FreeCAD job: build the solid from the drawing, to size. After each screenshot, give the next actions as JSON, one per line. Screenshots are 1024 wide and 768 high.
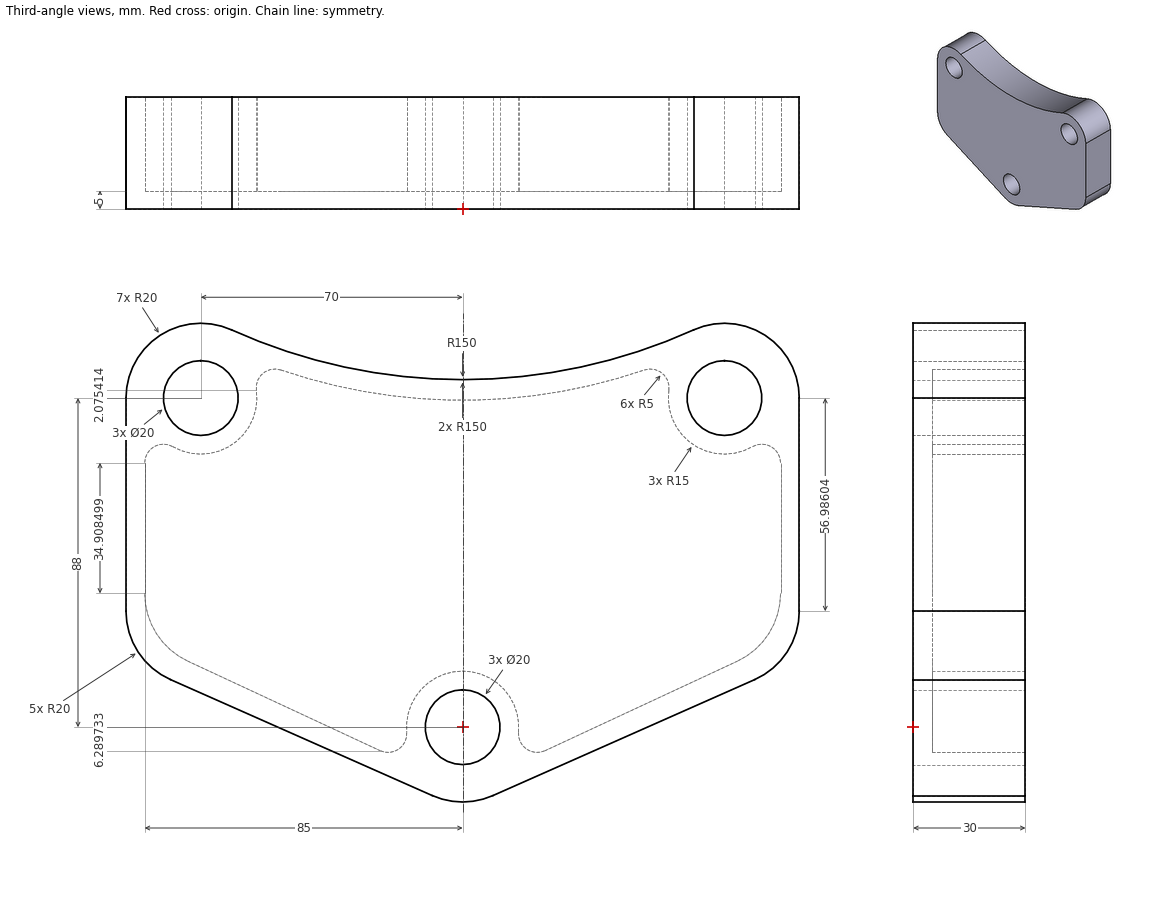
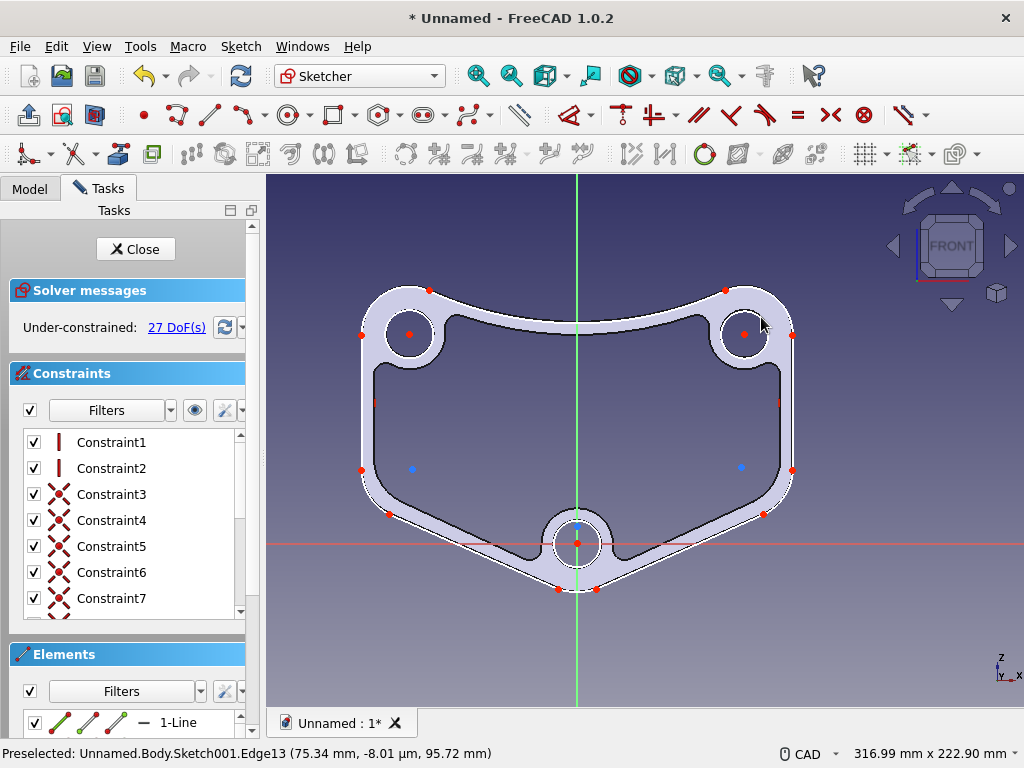
{"action": "left_click", "coordinate": [362, 376]}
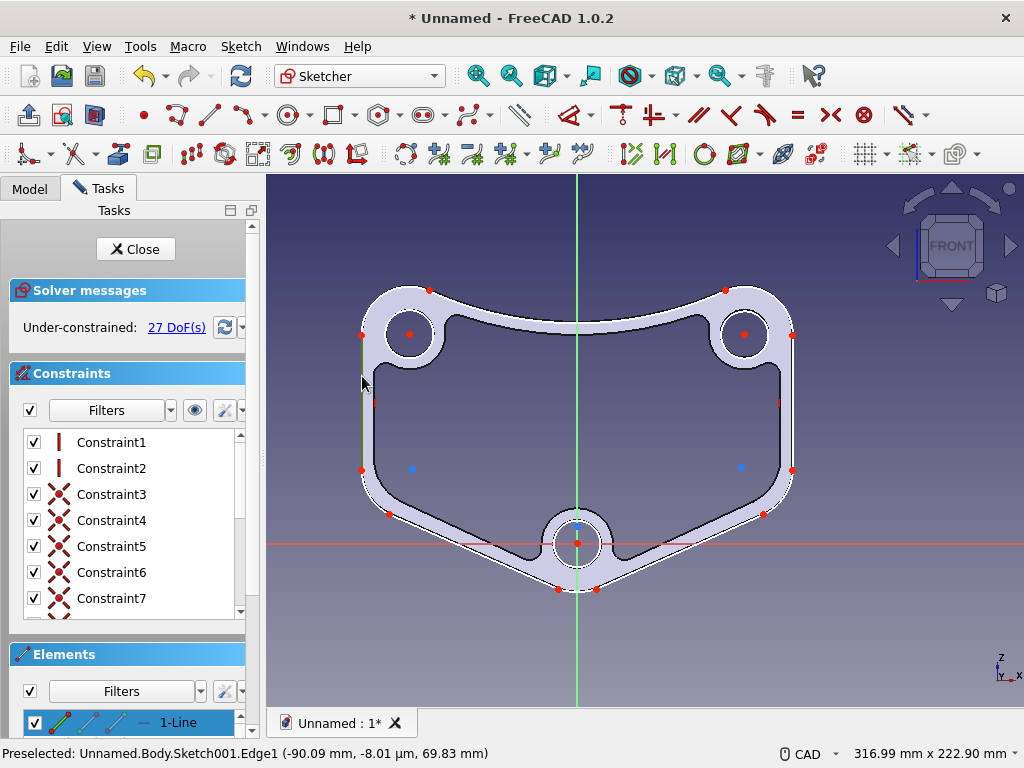
{"action": "left_click", "coordinate": [365, 487]}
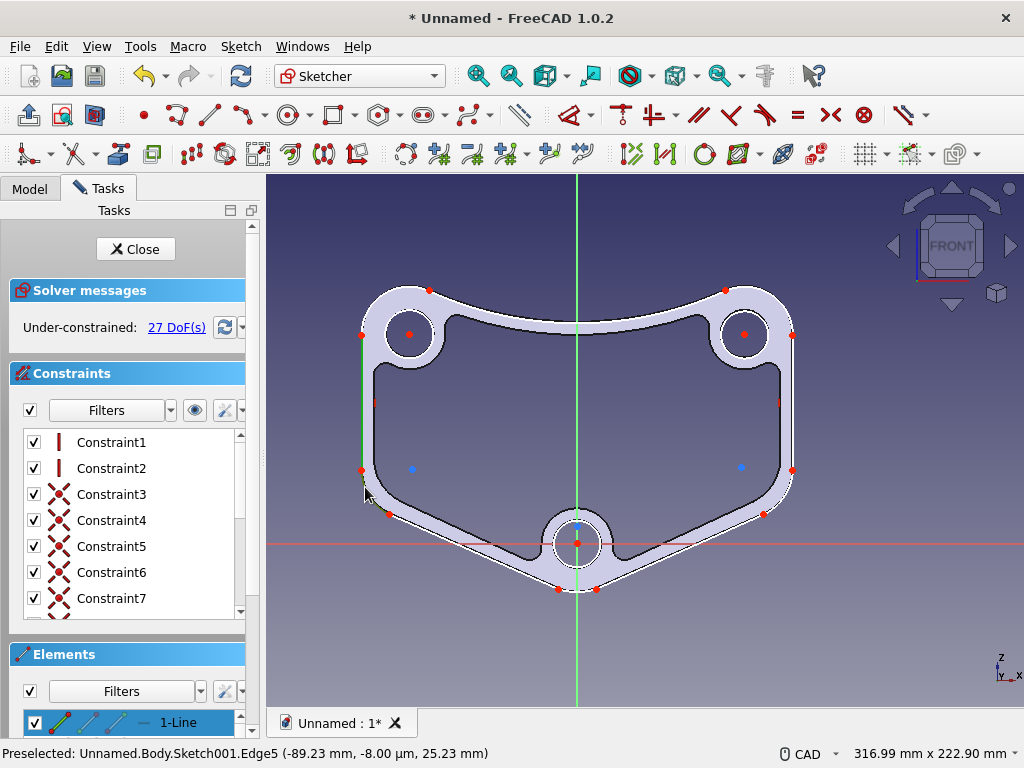
{"action": "left_click", "coordinate": [765, 116]}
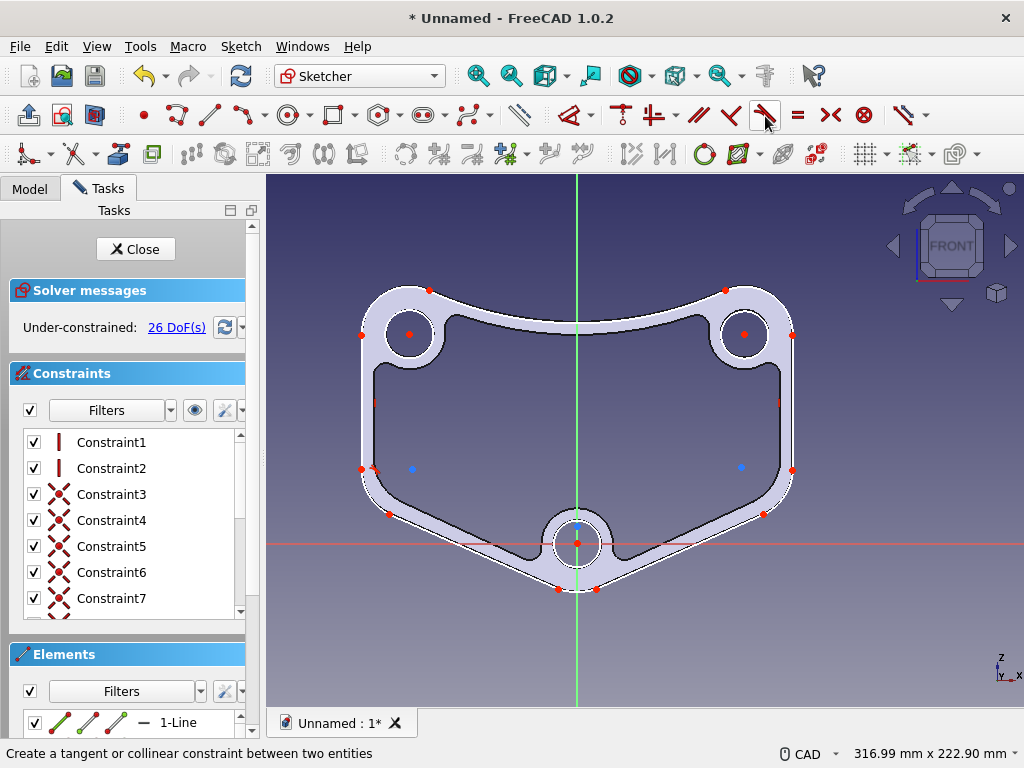
{"action": "left_click", "coordinate": [362, 375]}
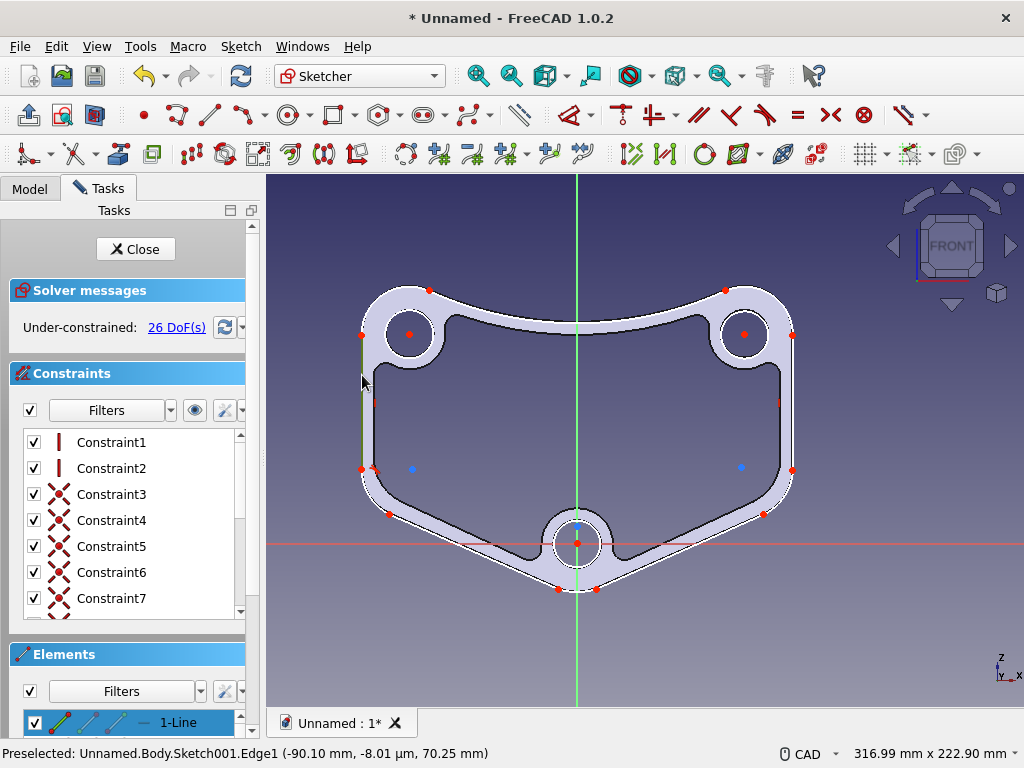
{"action": "left_click", "coordinate": [401, 287]}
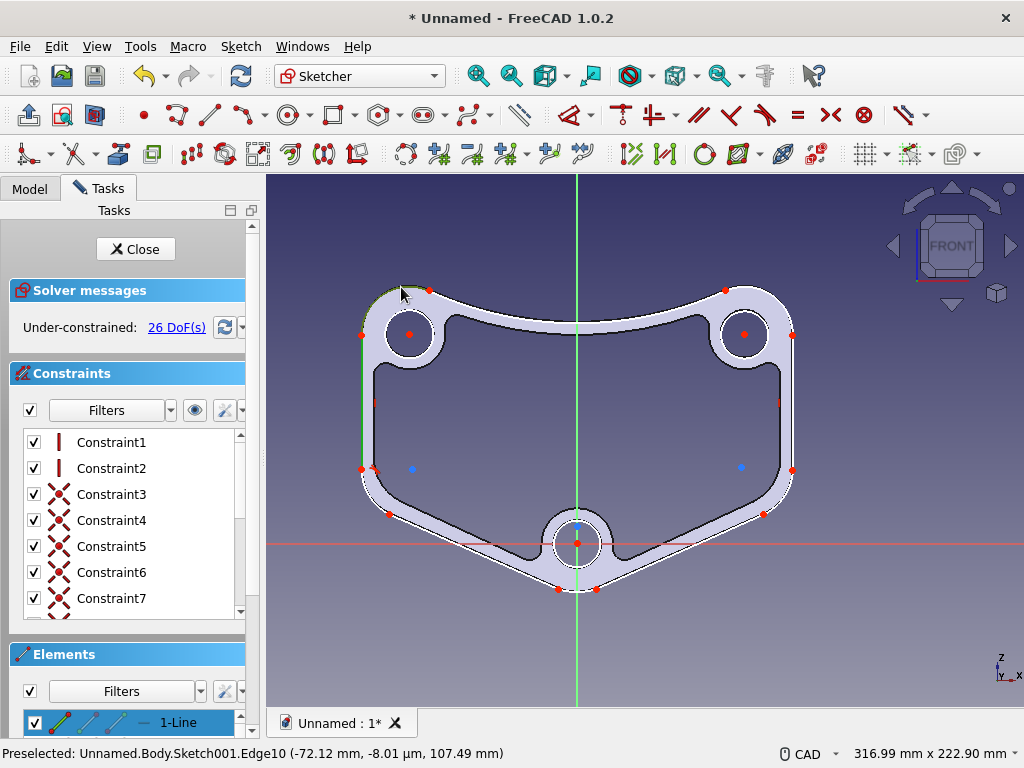
{"action": "left_click", "coordinate": [765, 116]}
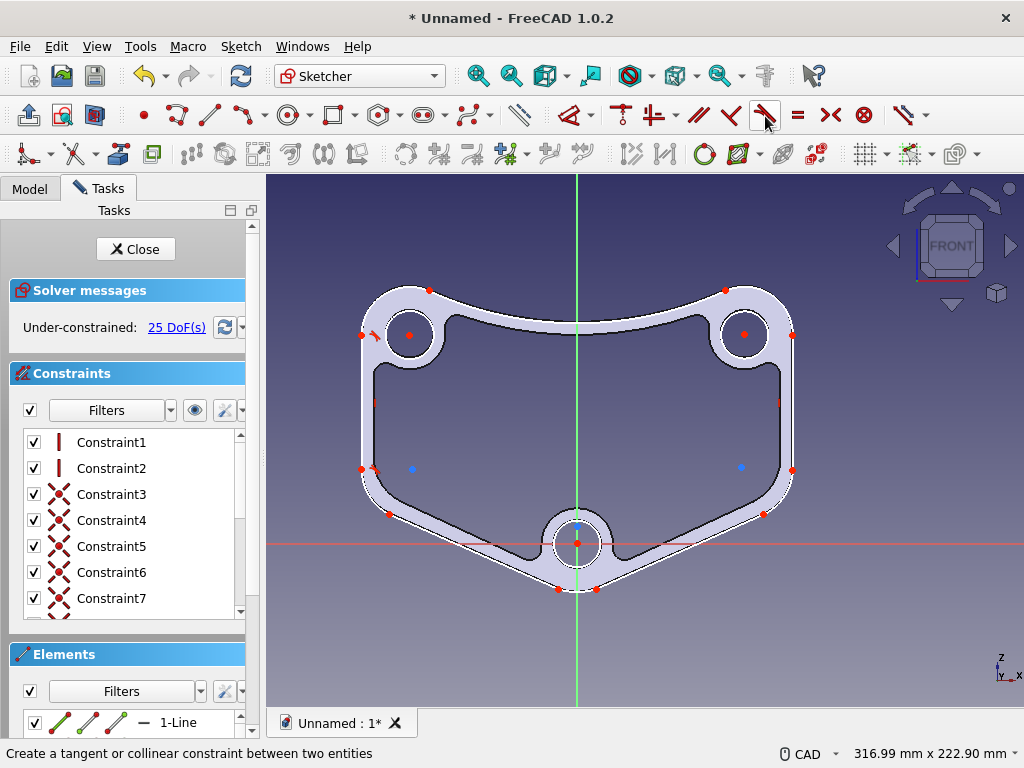
{"action": "left_click", "coordinate": [508, 567]}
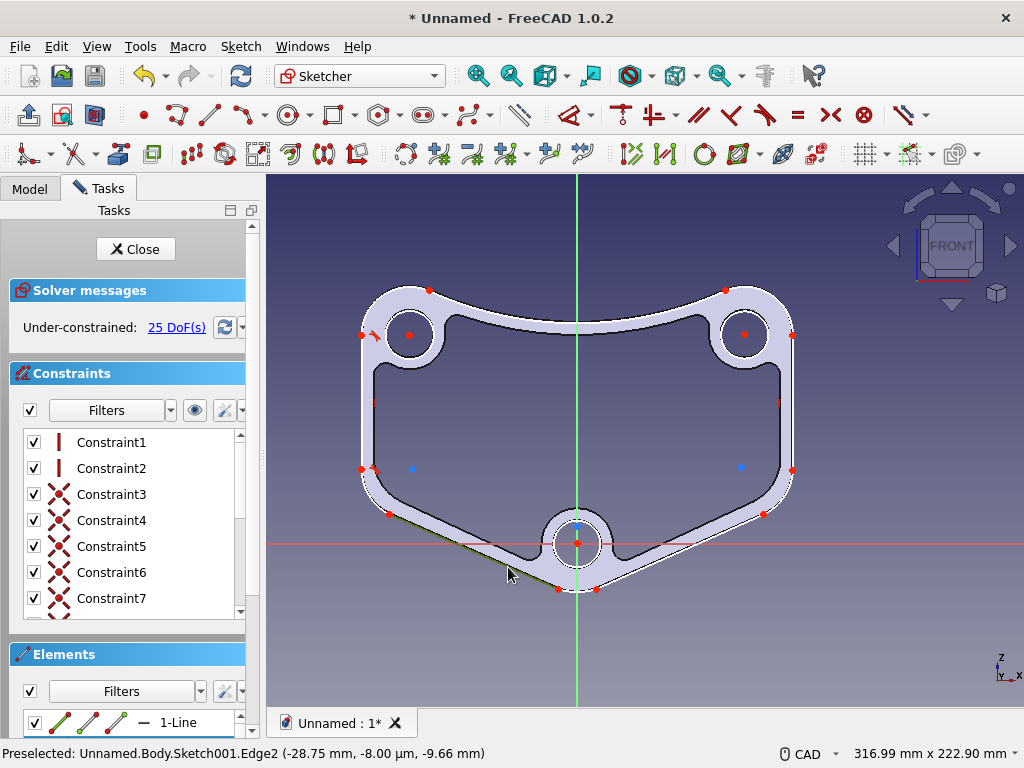
{"action": "left_click", "coordinate": [364, 486]}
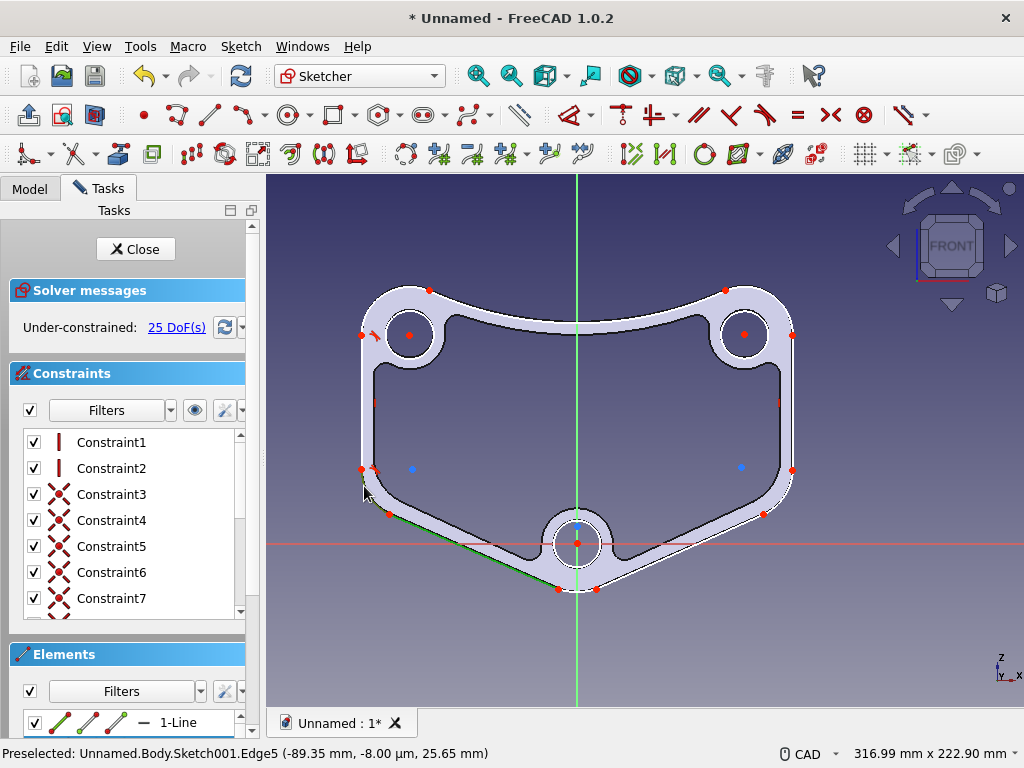
{"action": "left_click", "coordinate": [765, 116]}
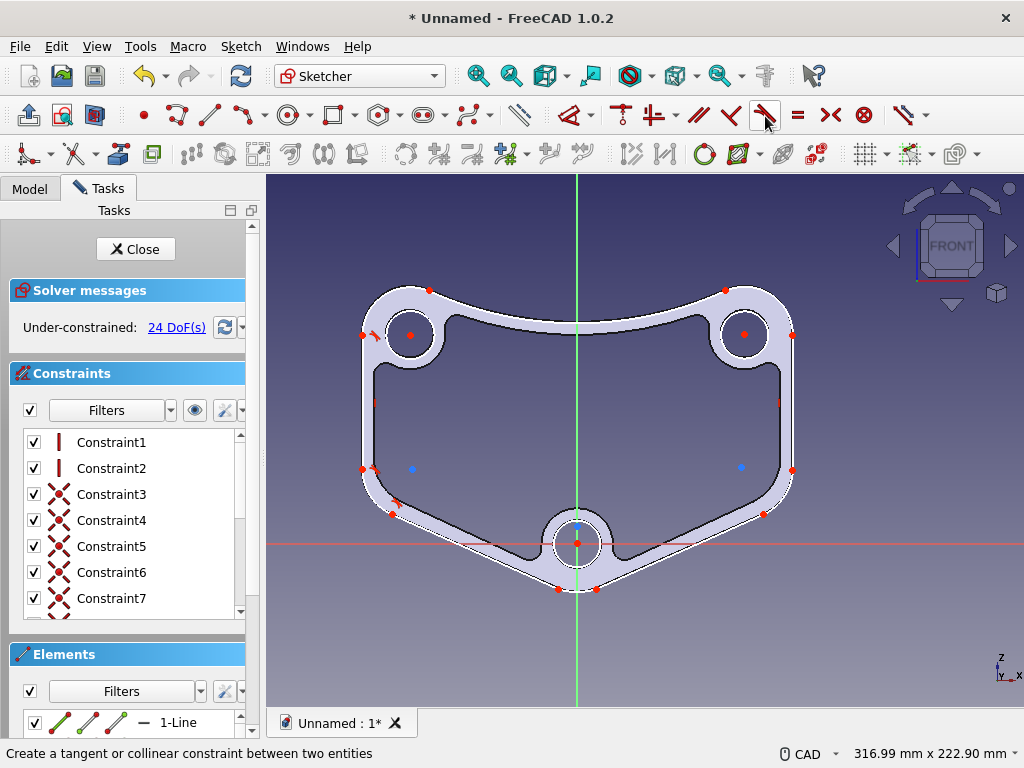
{"action": "left_click", "coordinate": [508, 567]}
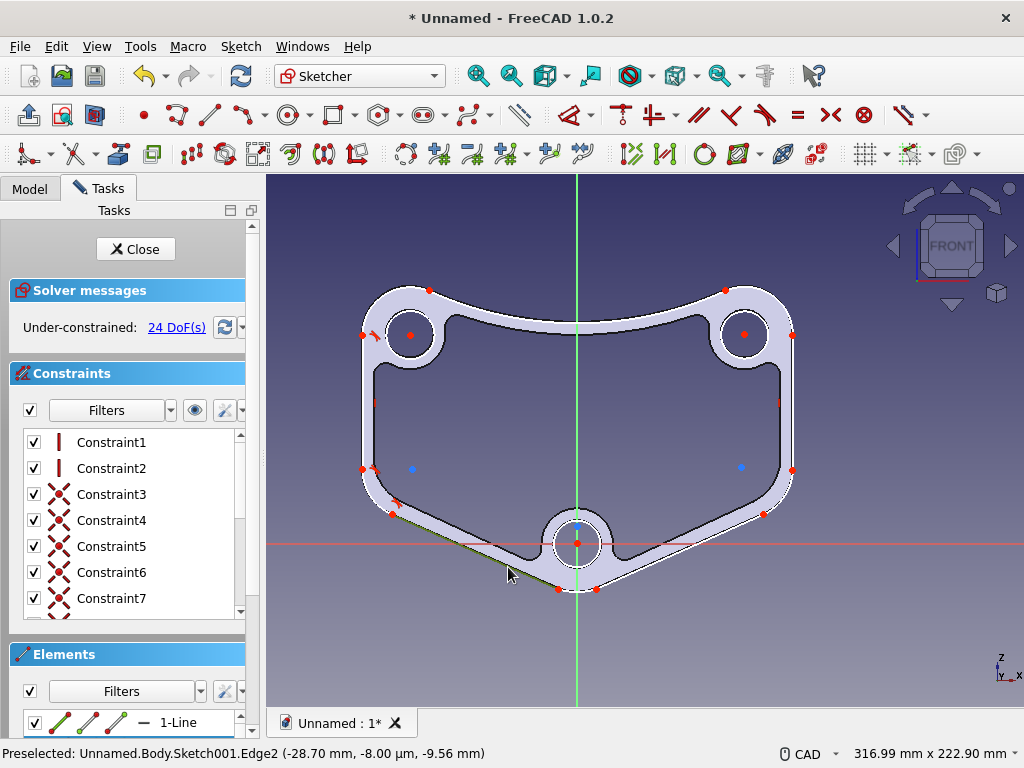
{"action": "left_click", "coordinate": [577, 592]}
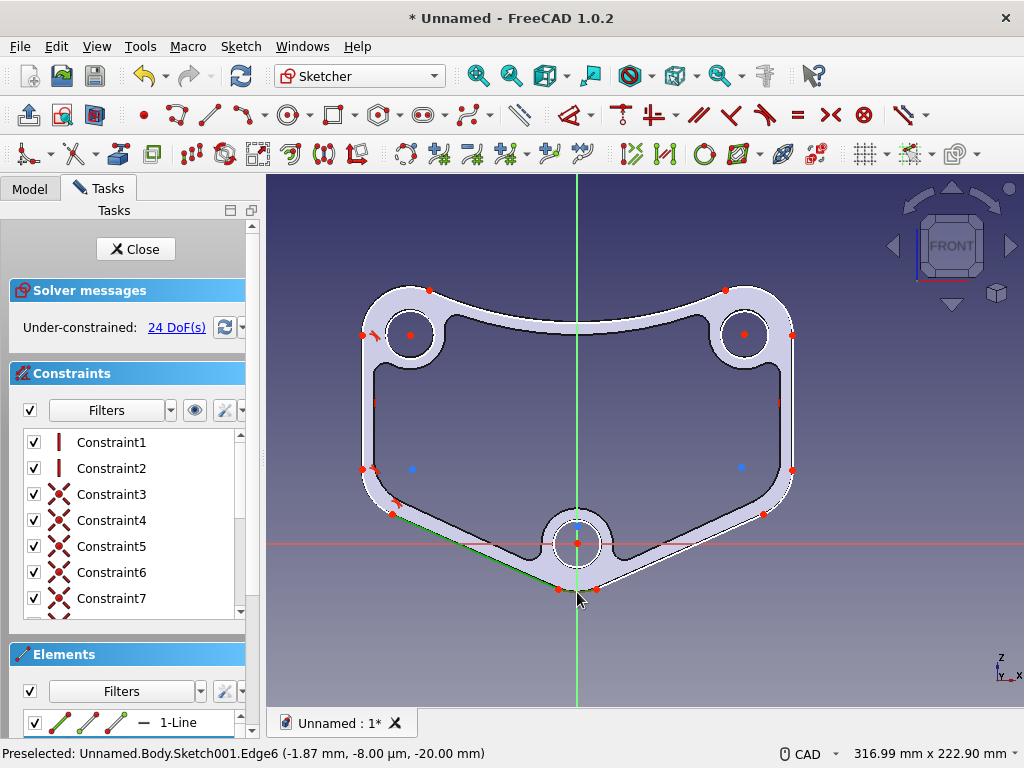
{"action": "left_click", "coordinate": [765, 116]}